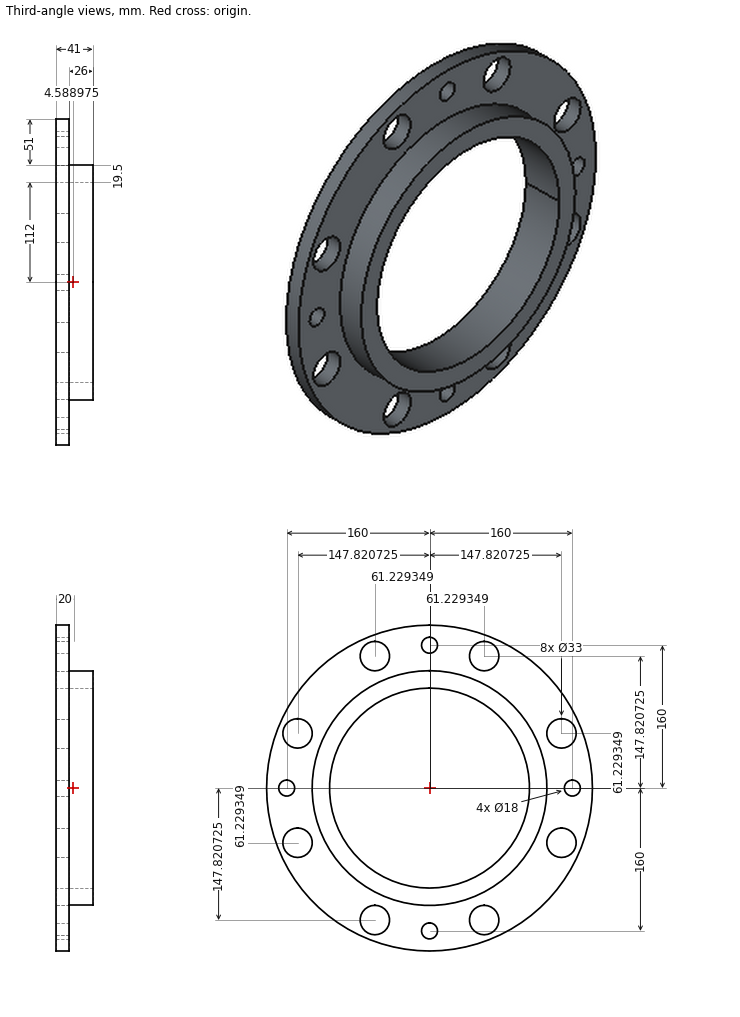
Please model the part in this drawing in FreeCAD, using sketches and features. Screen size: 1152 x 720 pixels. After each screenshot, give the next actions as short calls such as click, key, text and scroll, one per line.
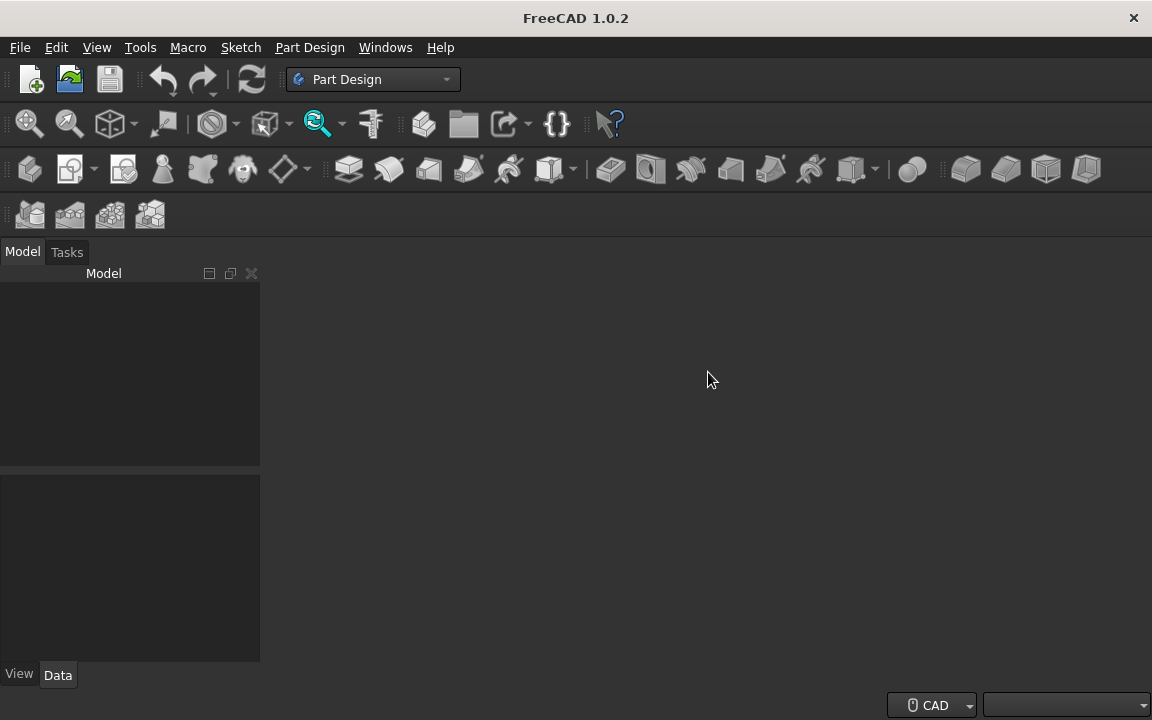
click(30, 80)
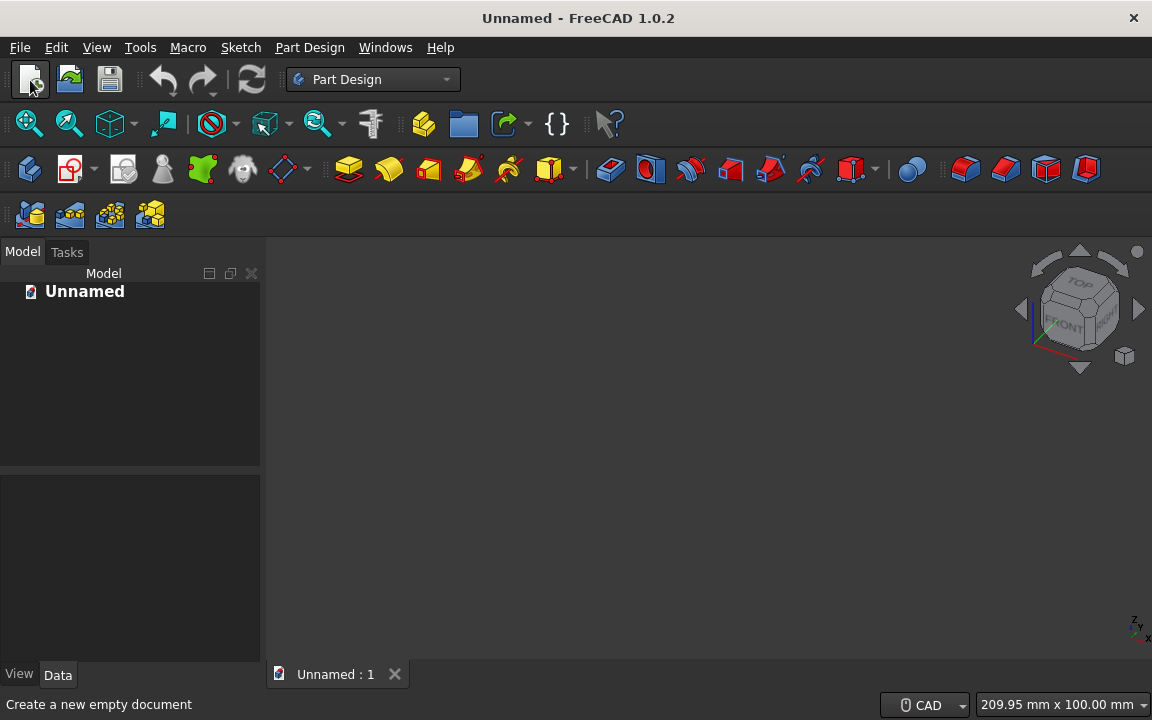
click(70, 170)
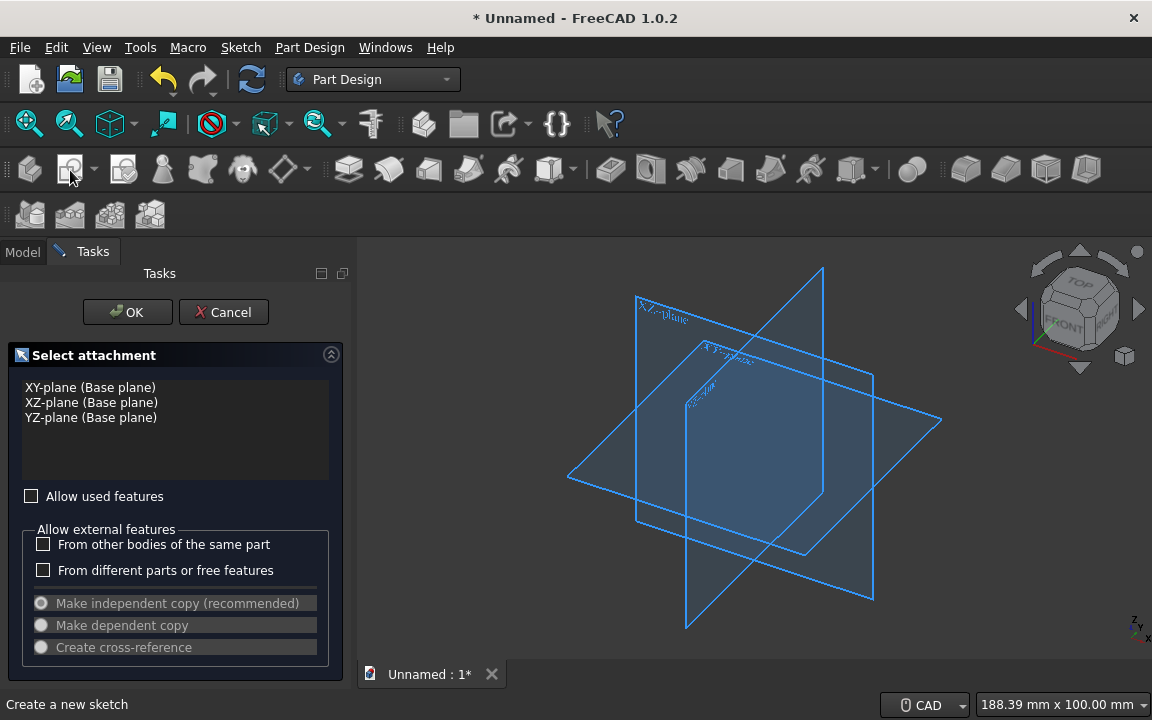
click(82, 388)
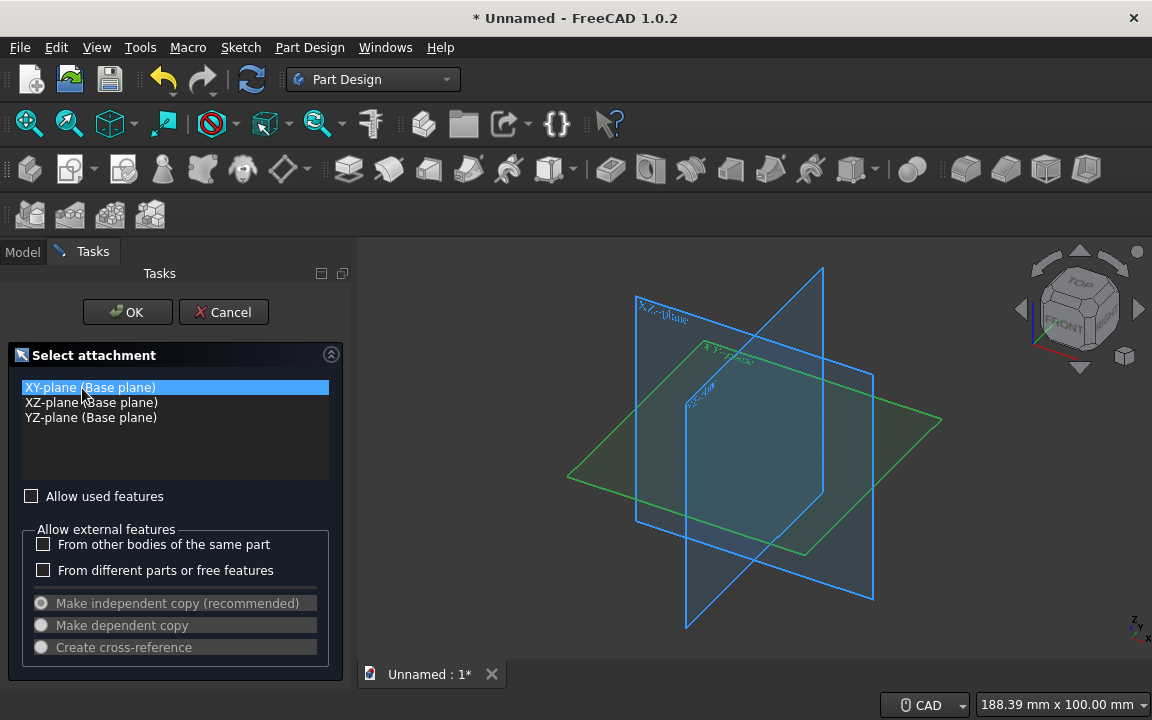
click(128, 312)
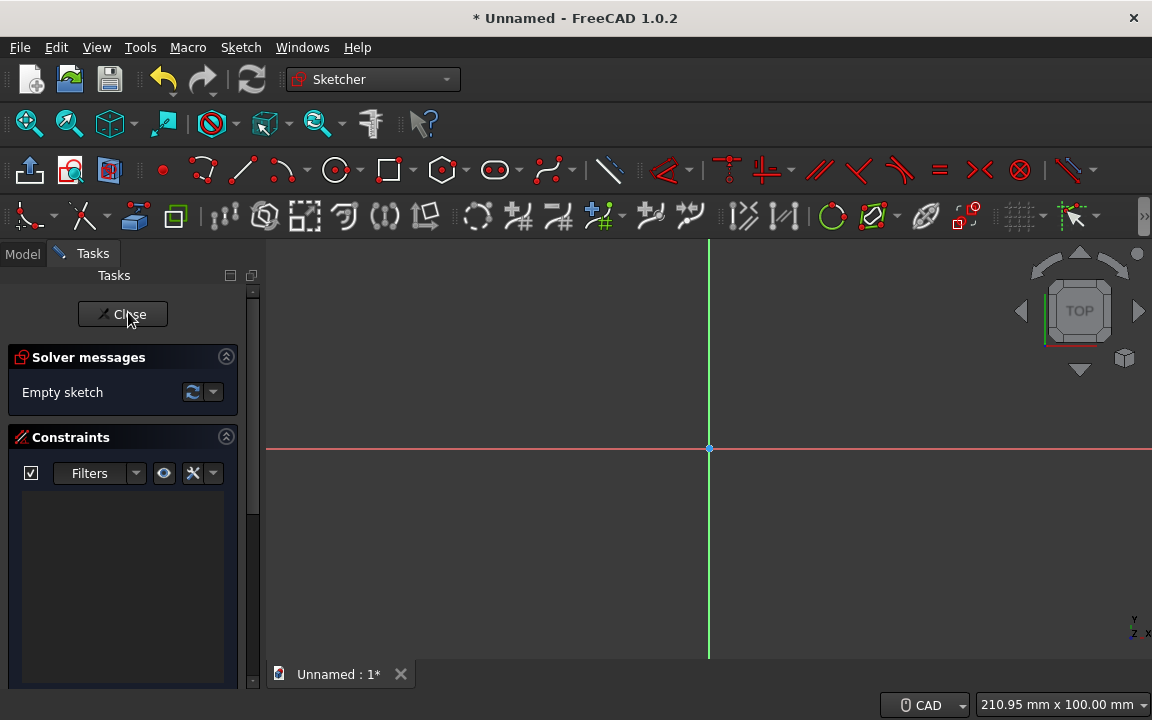
scroll(640, 449, down, 5)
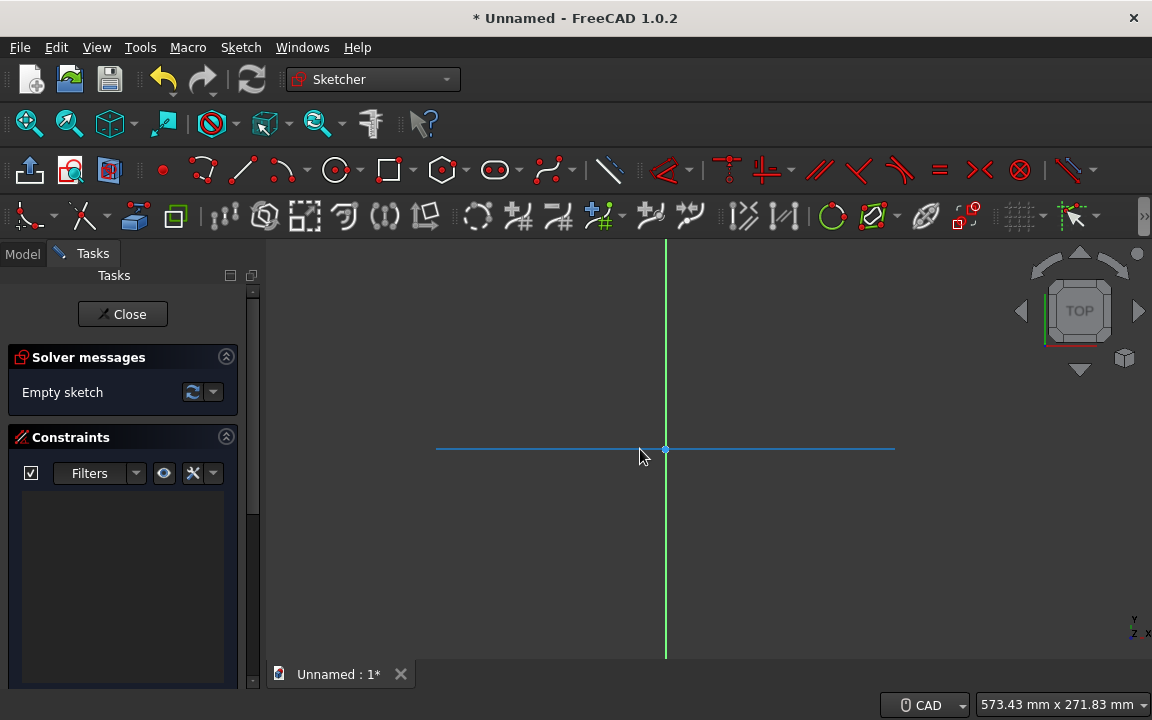
scroll(640, 449, down, 5)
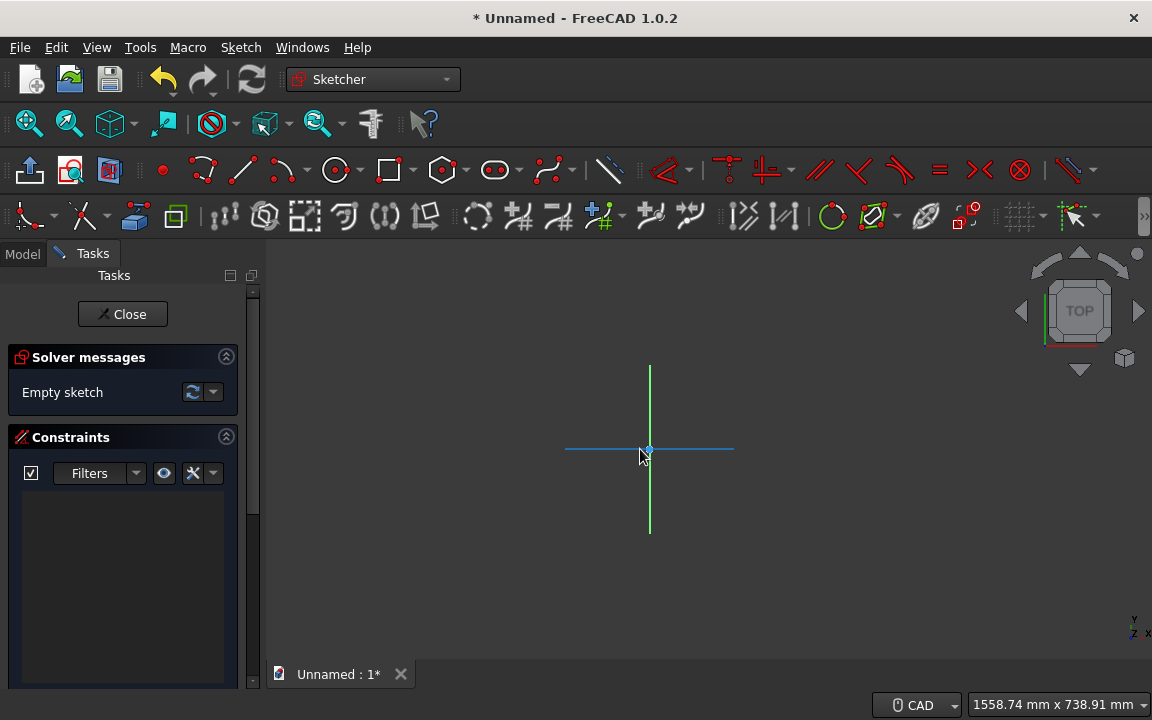
scroll(652, 349, up, 9)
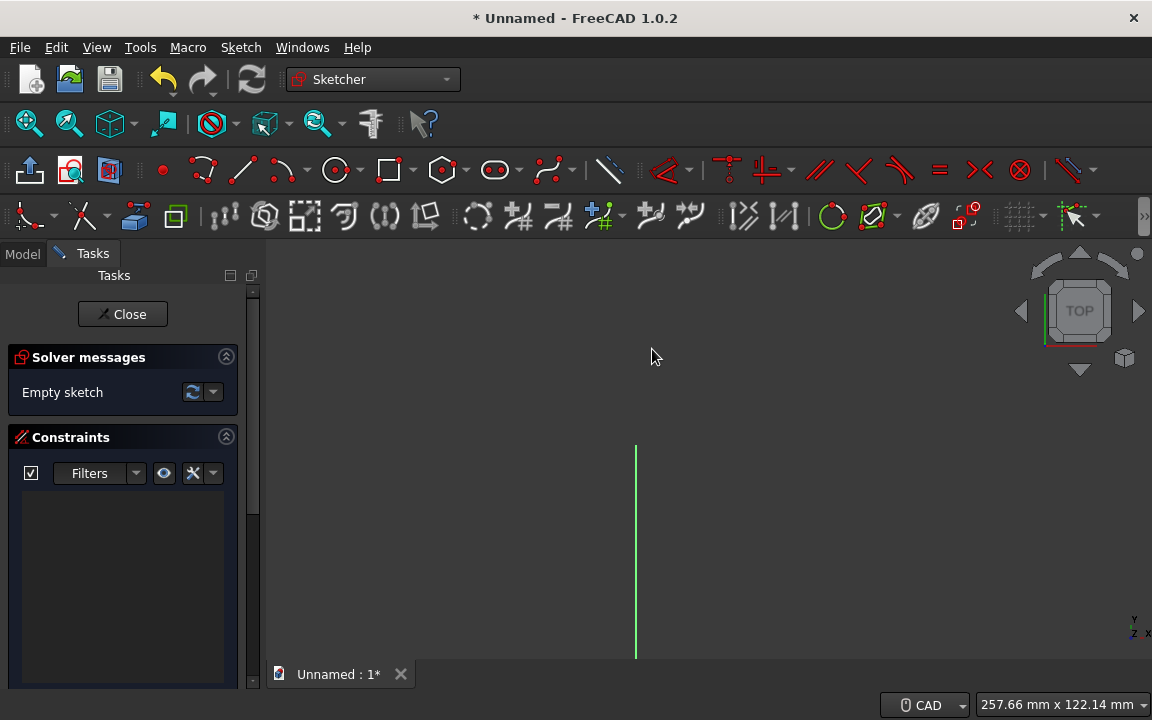
click(204, 170)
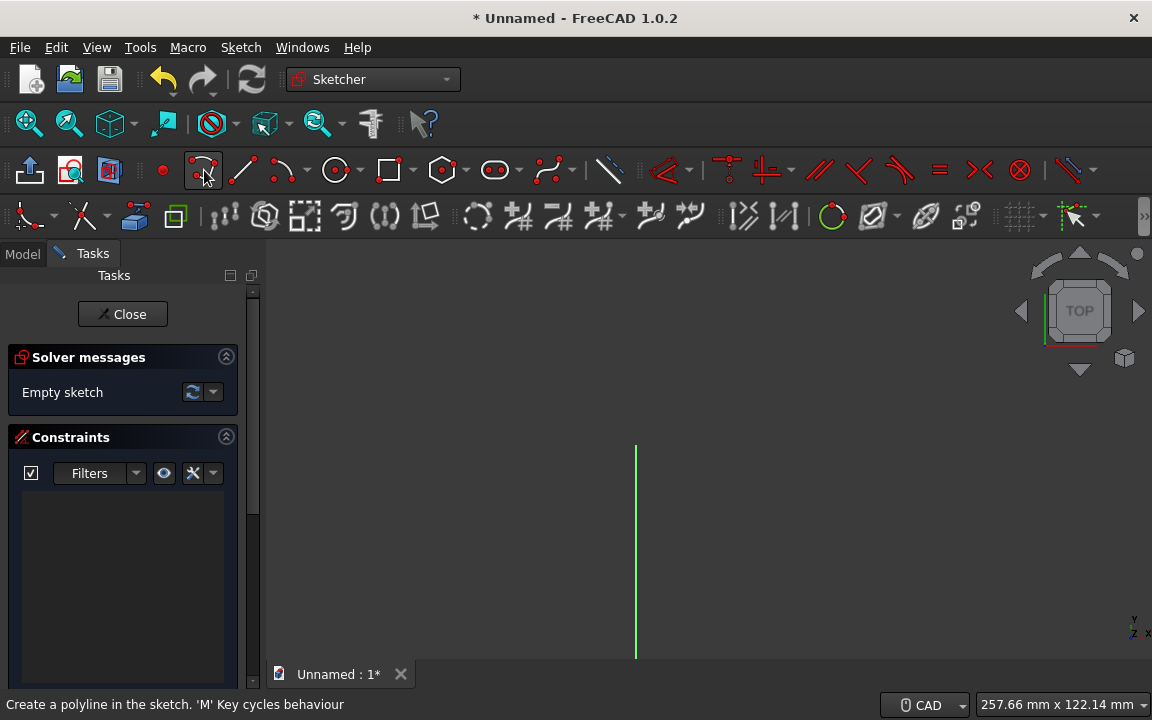
click(569, 570)
click(710, 570)
click(710, 503)
click(620, 503)
click(620, 328)
click(569, 328)
click(569, 571)
key(Escape)
key(Escape)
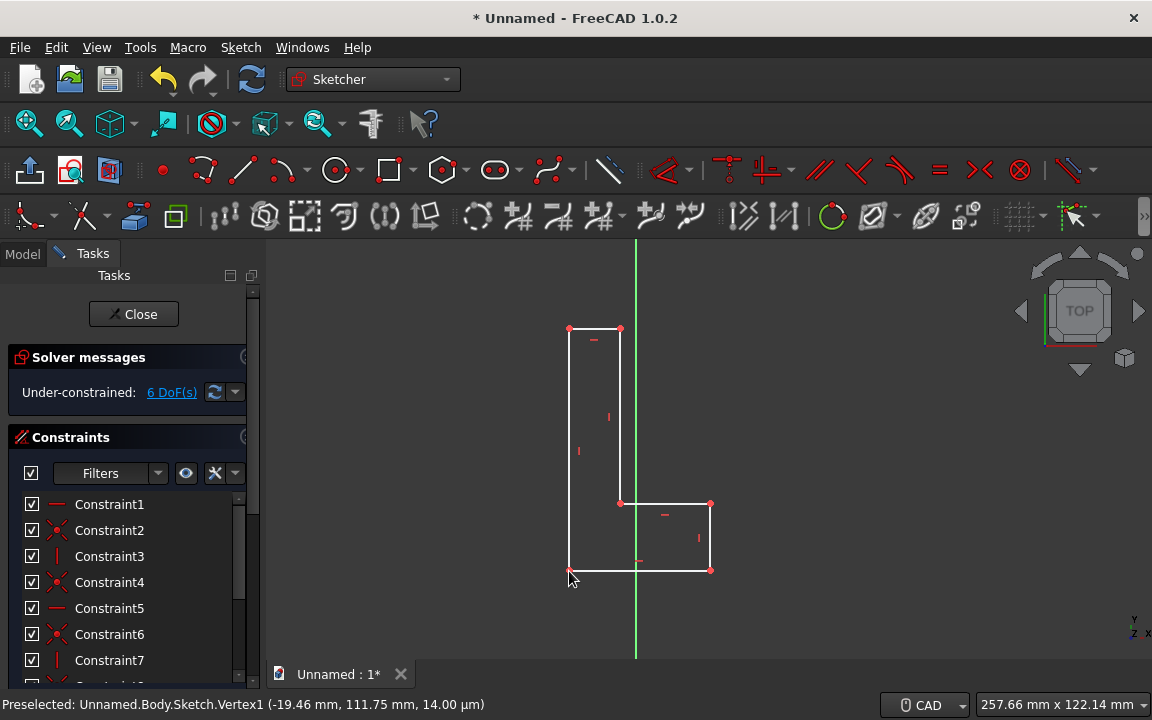
click(664, 170)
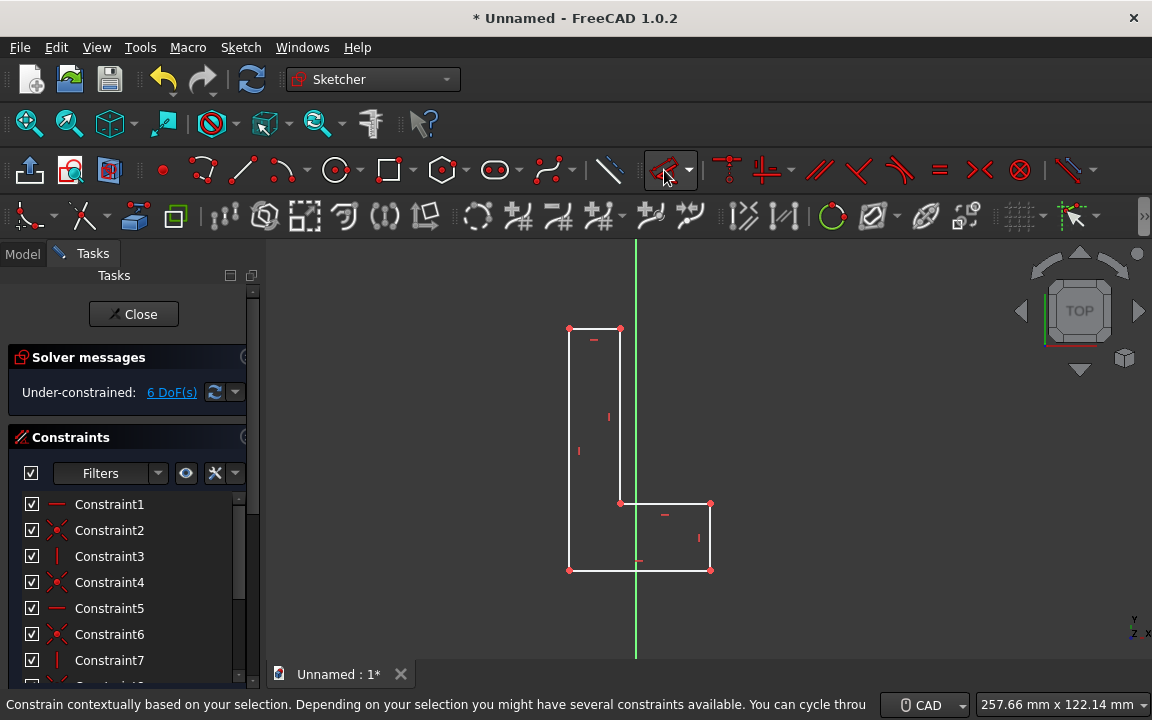
click(611, 571)
click(607, 605)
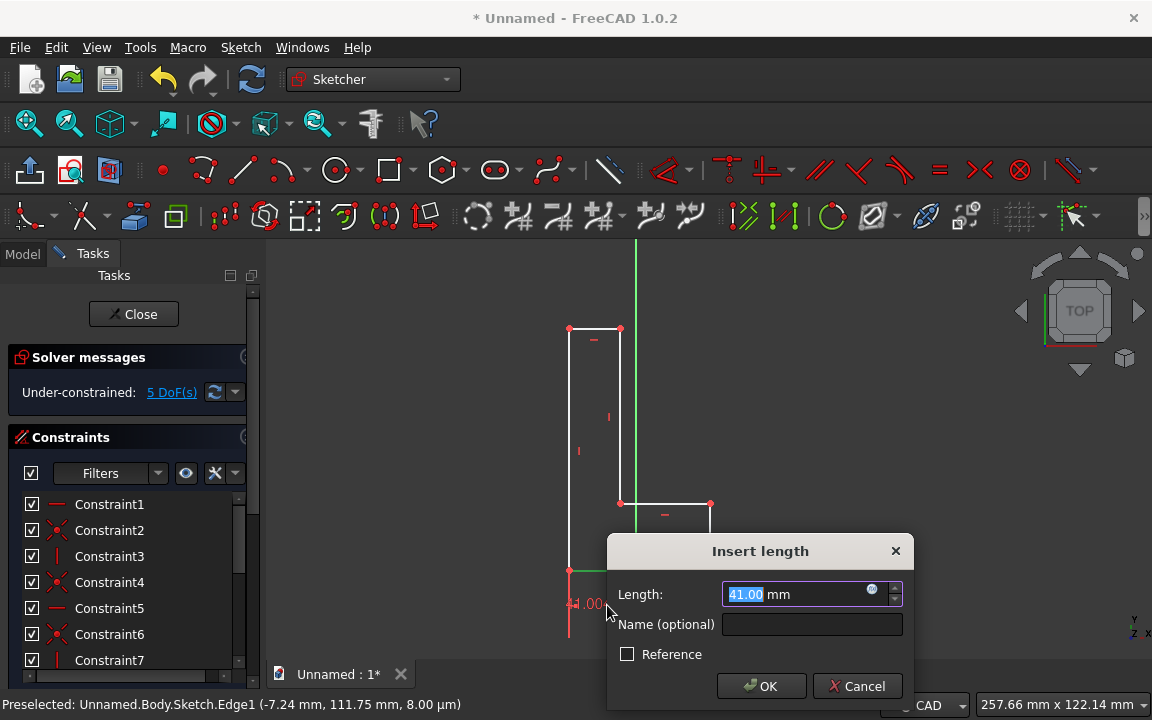
text(41)
key(Return)